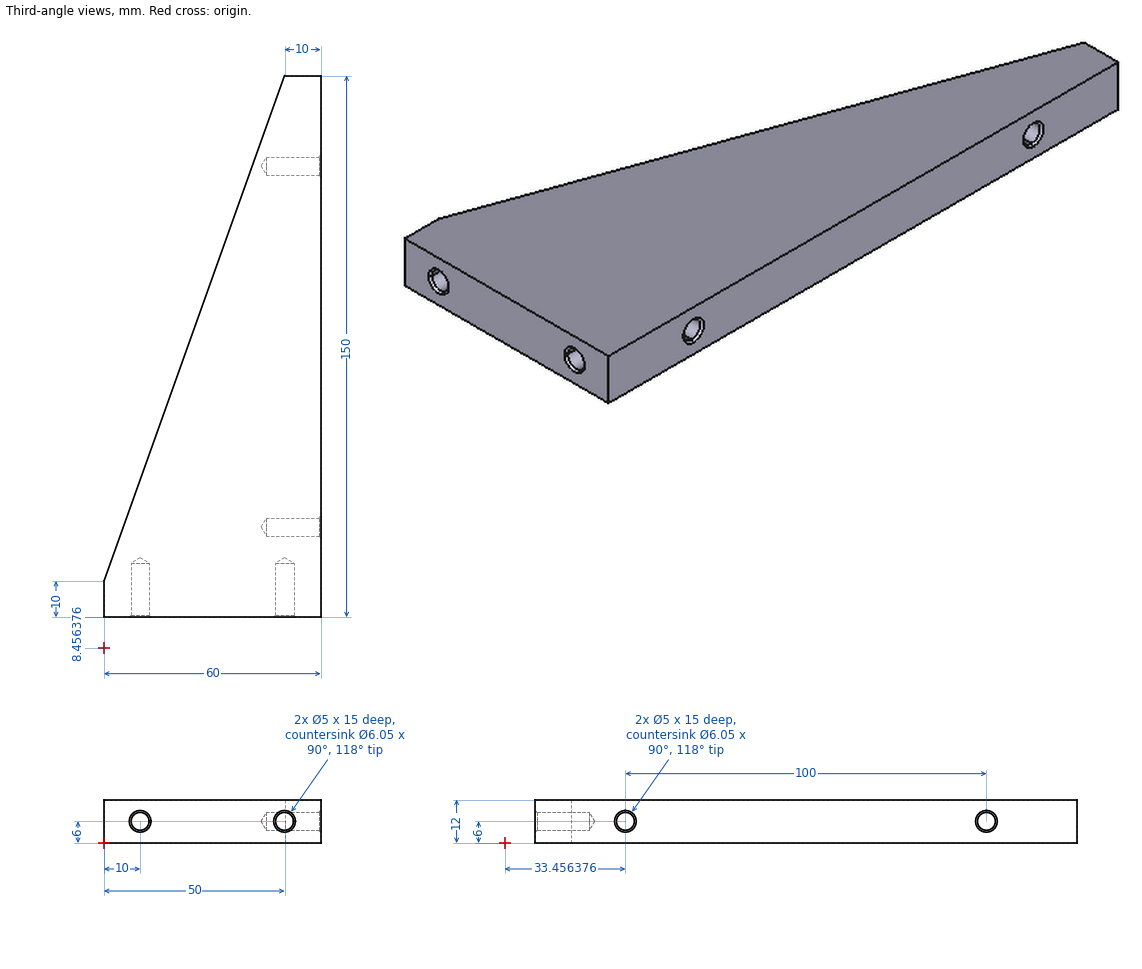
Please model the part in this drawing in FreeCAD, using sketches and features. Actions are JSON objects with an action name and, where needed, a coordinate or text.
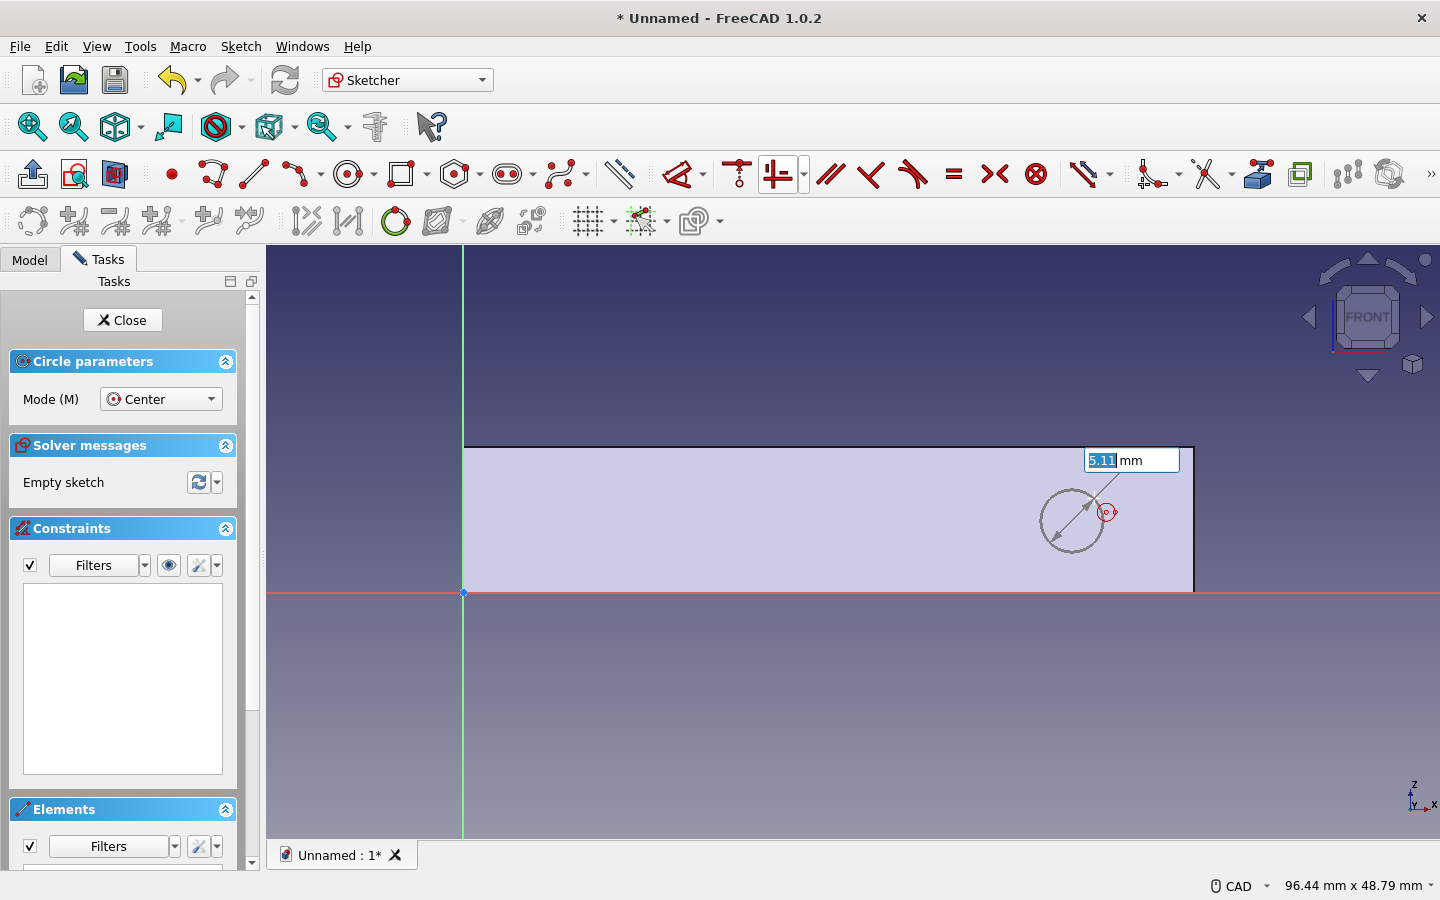
{"action": "type", "text": "5"}
{"action": "key", "text": "Return"}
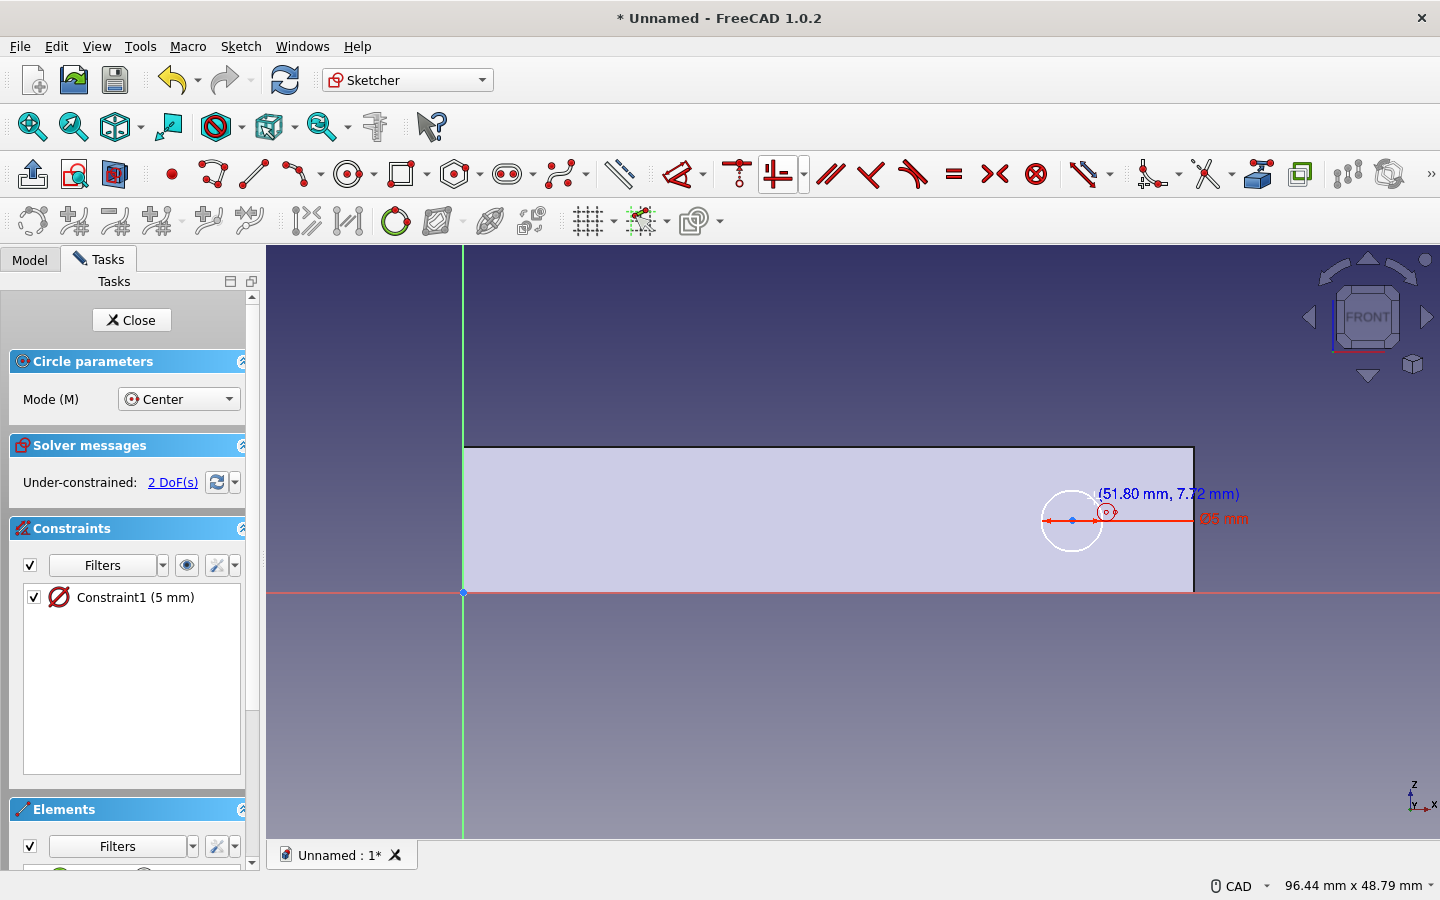
{"action": "left_click", "coordinate": [585, 520]}
{"action": "mouse_move", "coordinate": [607, 498]}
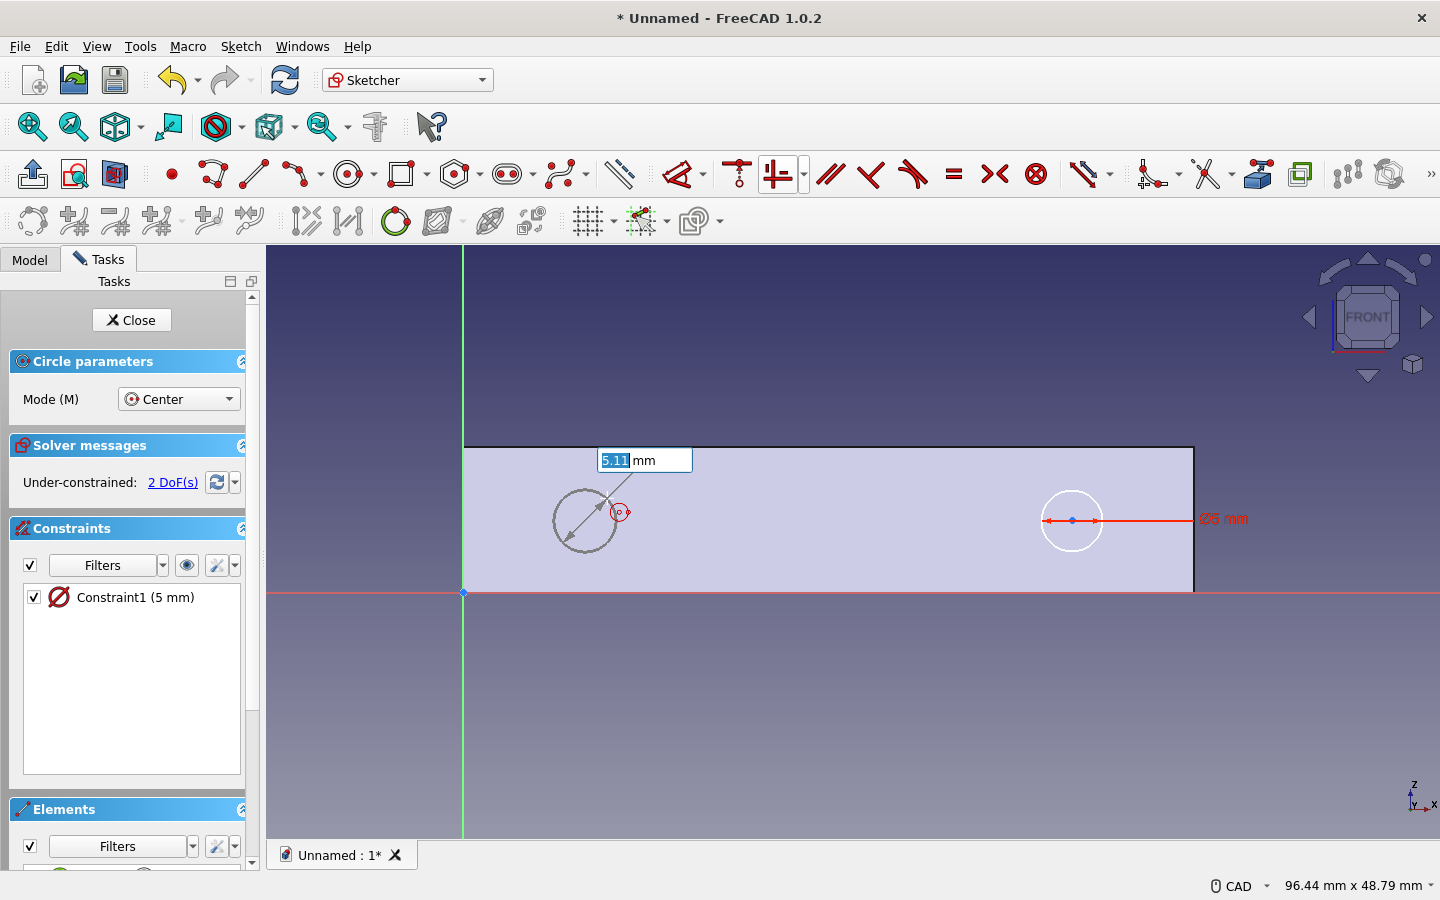
{"action": "type", "text": "5"}
{"action": "key", "text": "Return"}
{"action": "key", "text": "Escape"}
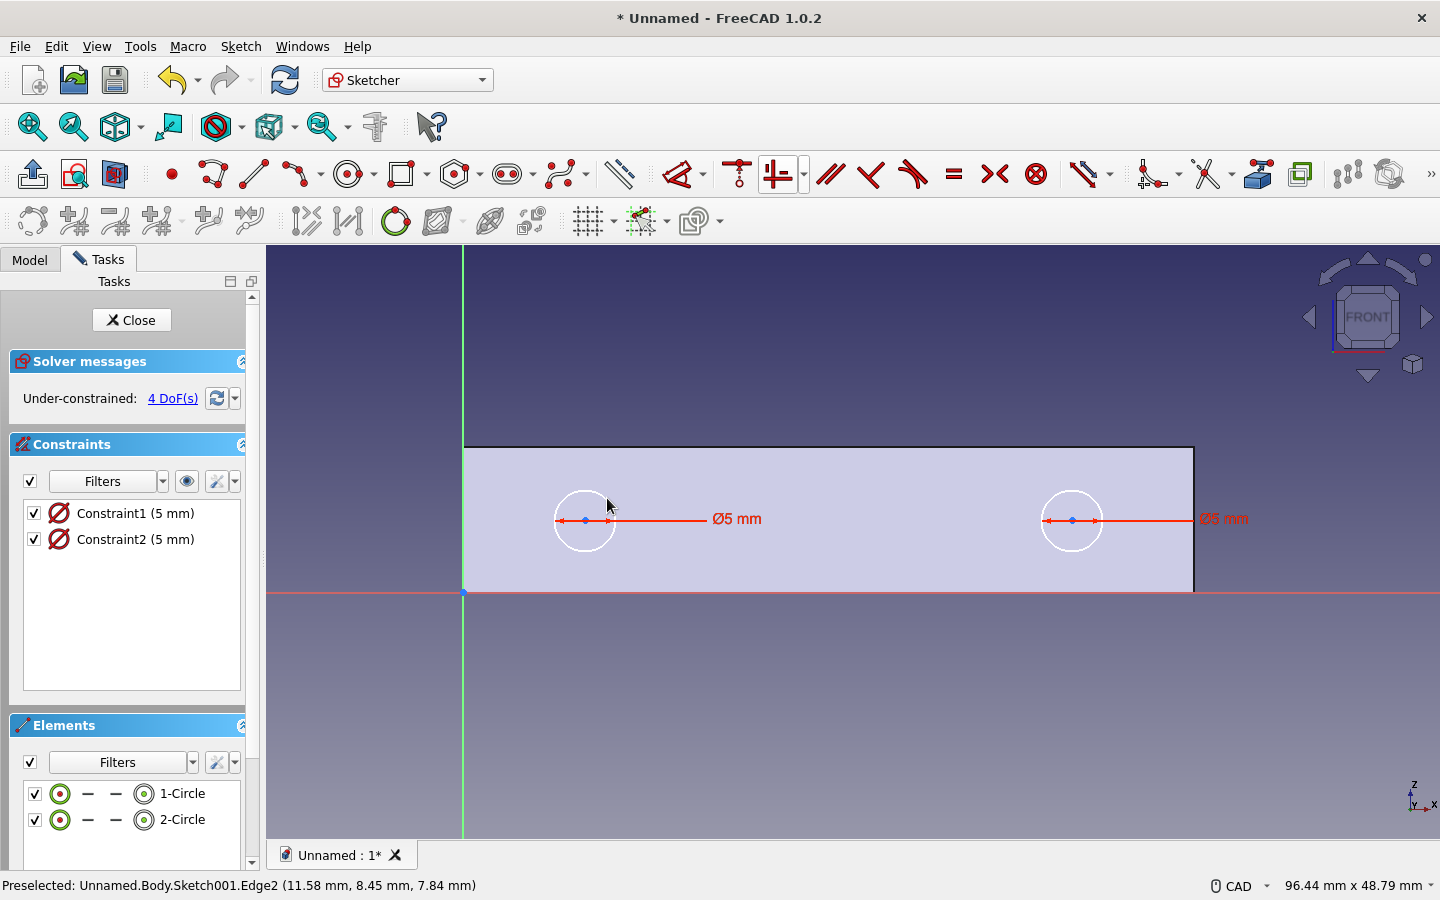
{"action": "left_click", "coordinate": [1072, 521]}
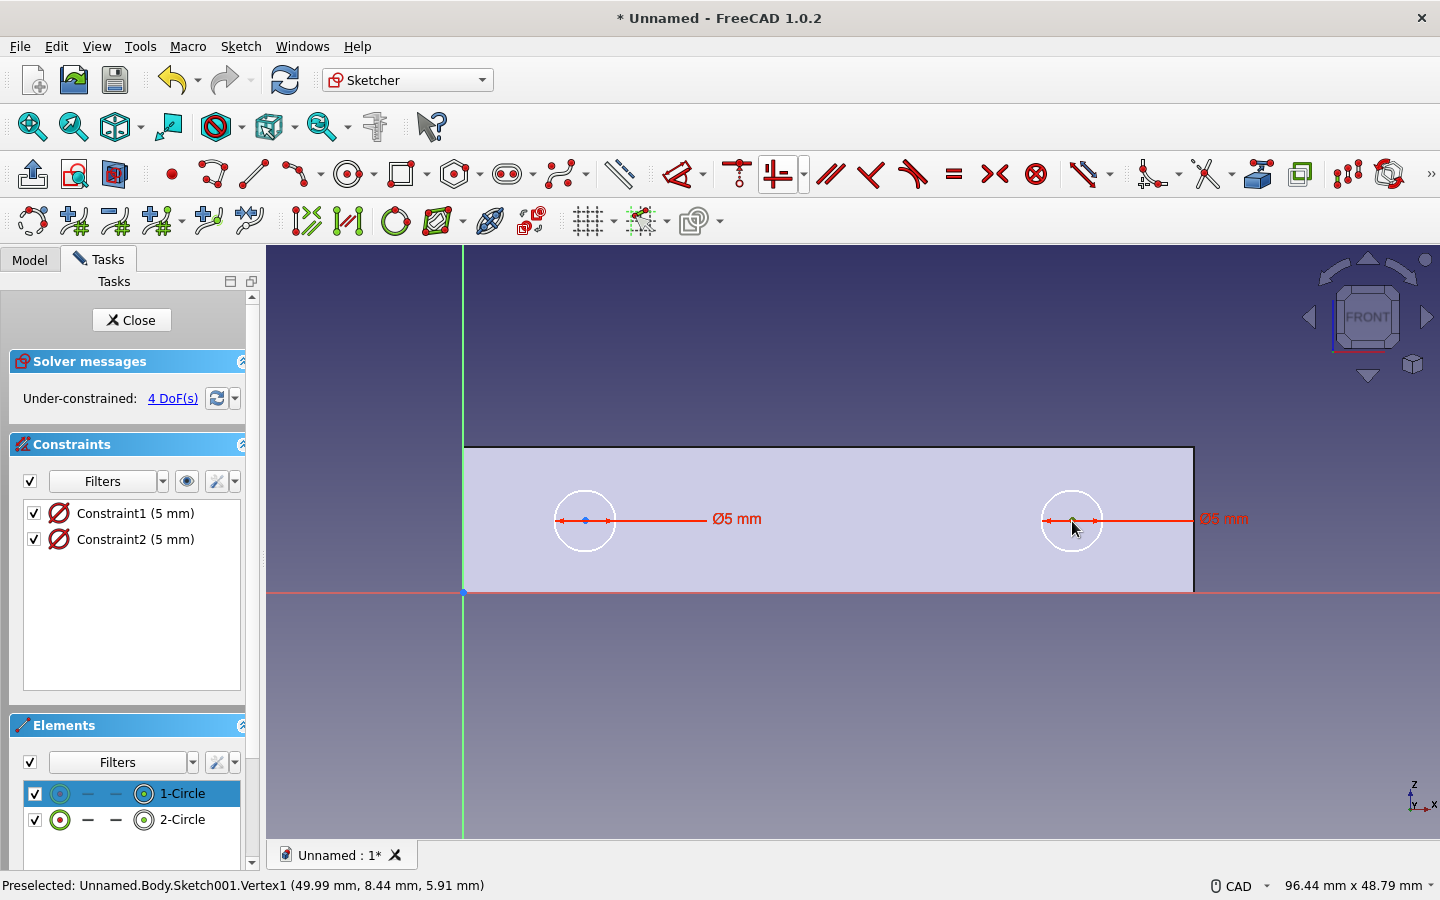
{"action": "left_click", "coordinate": [585, 521]}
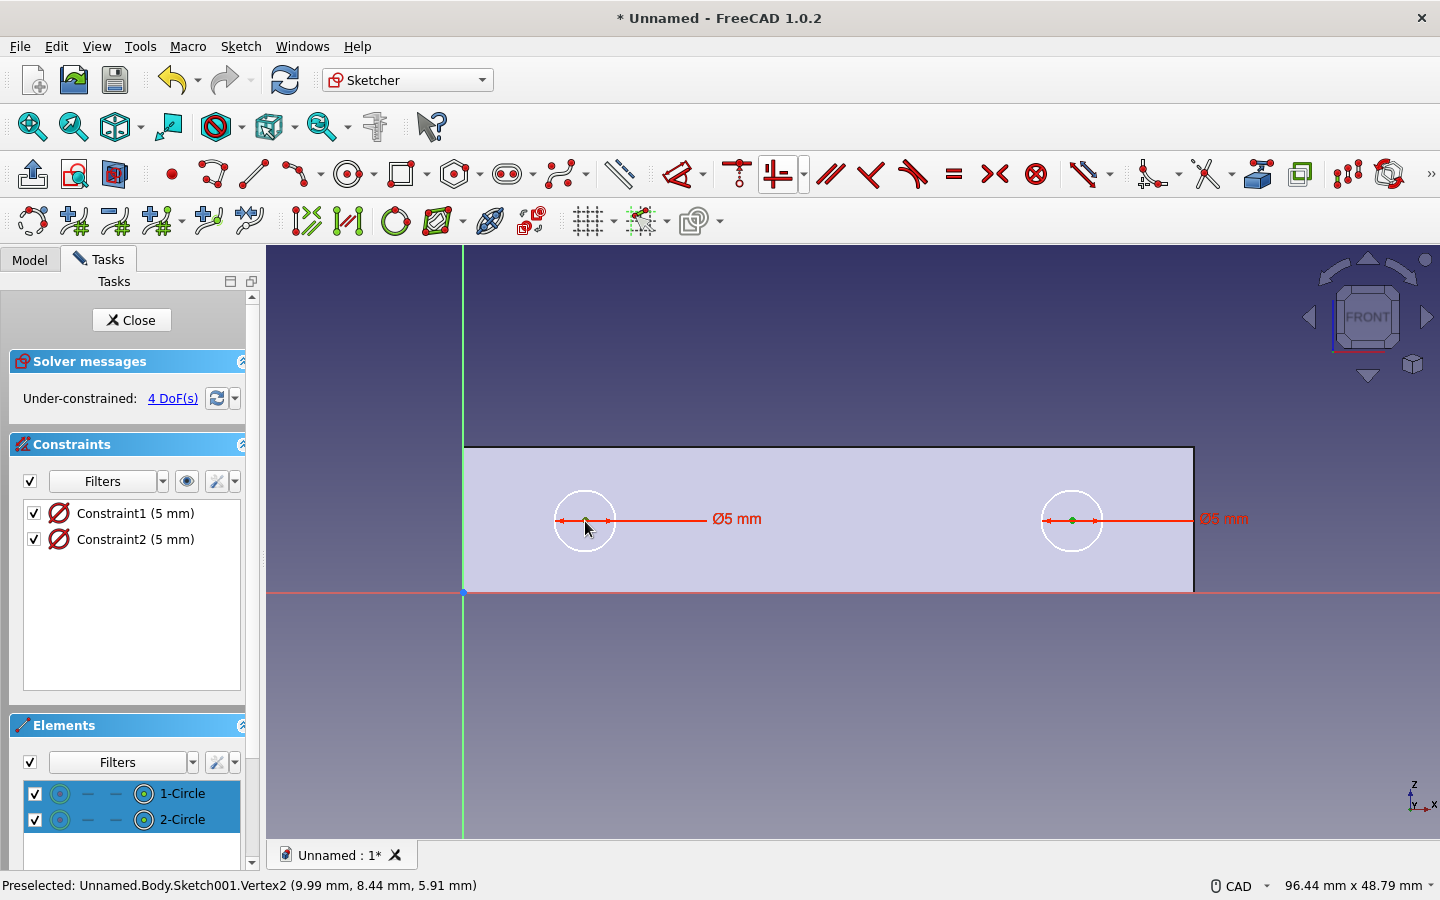
{"action": "left_click", "coordinate": [804, 174]}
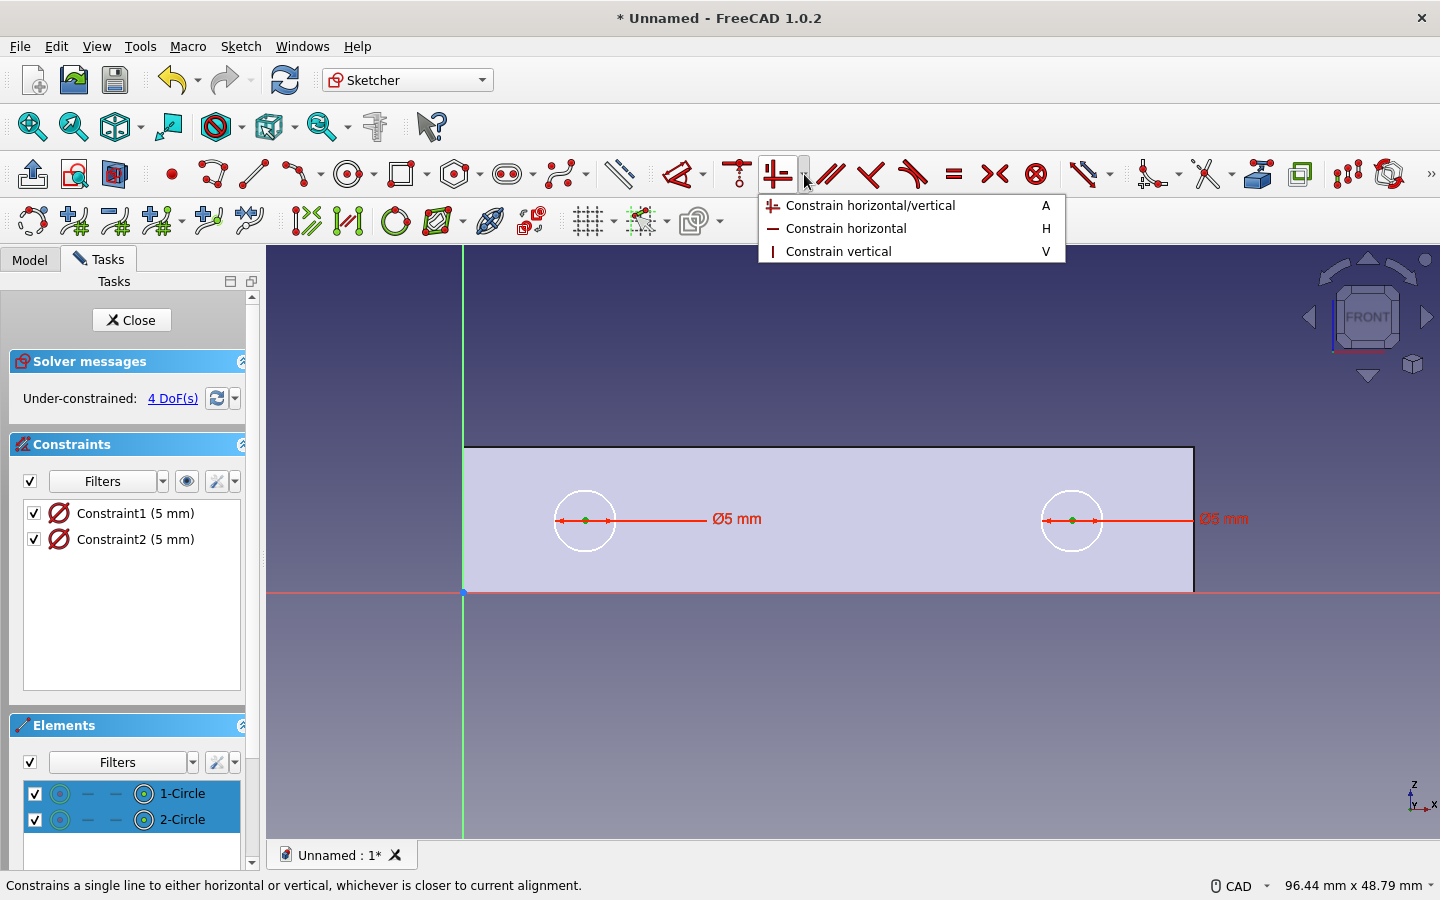
{"action": "left_click", "coordinate": [912, 228]}